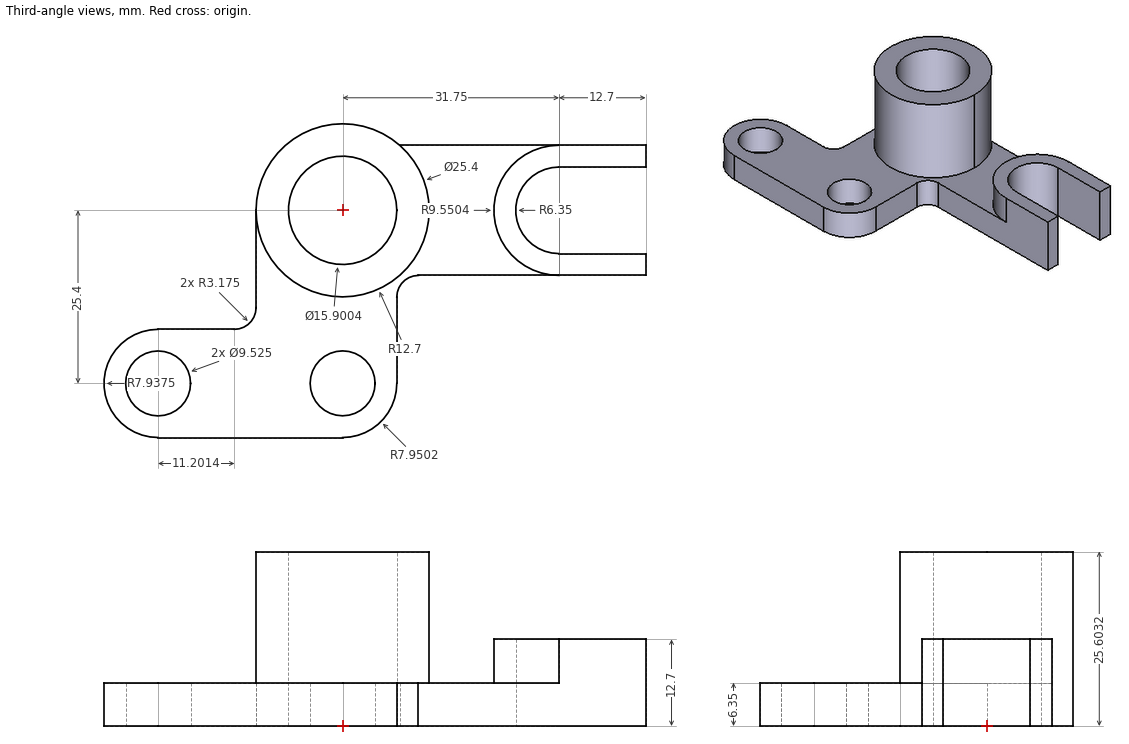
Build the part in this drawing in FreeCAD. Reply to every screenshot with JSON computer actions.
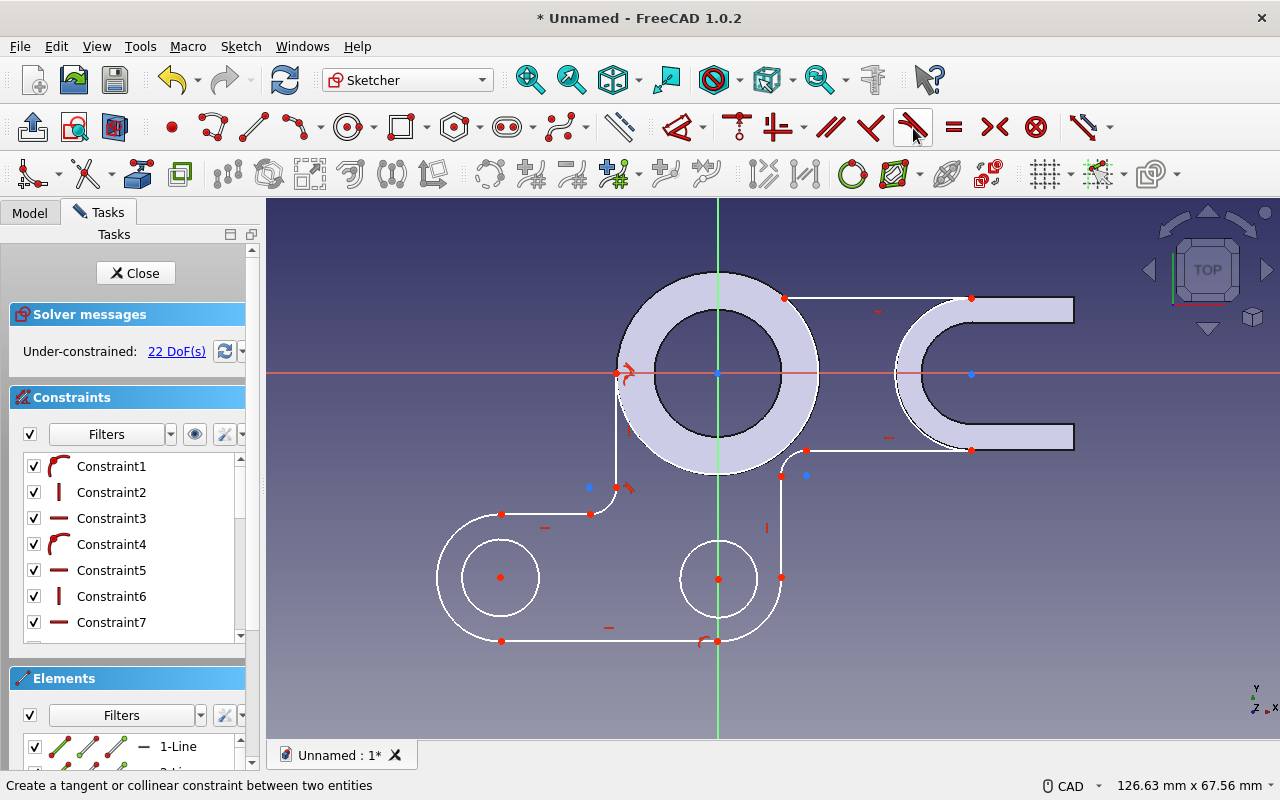
{"action": "left_click", "coordinate": [564, 514]}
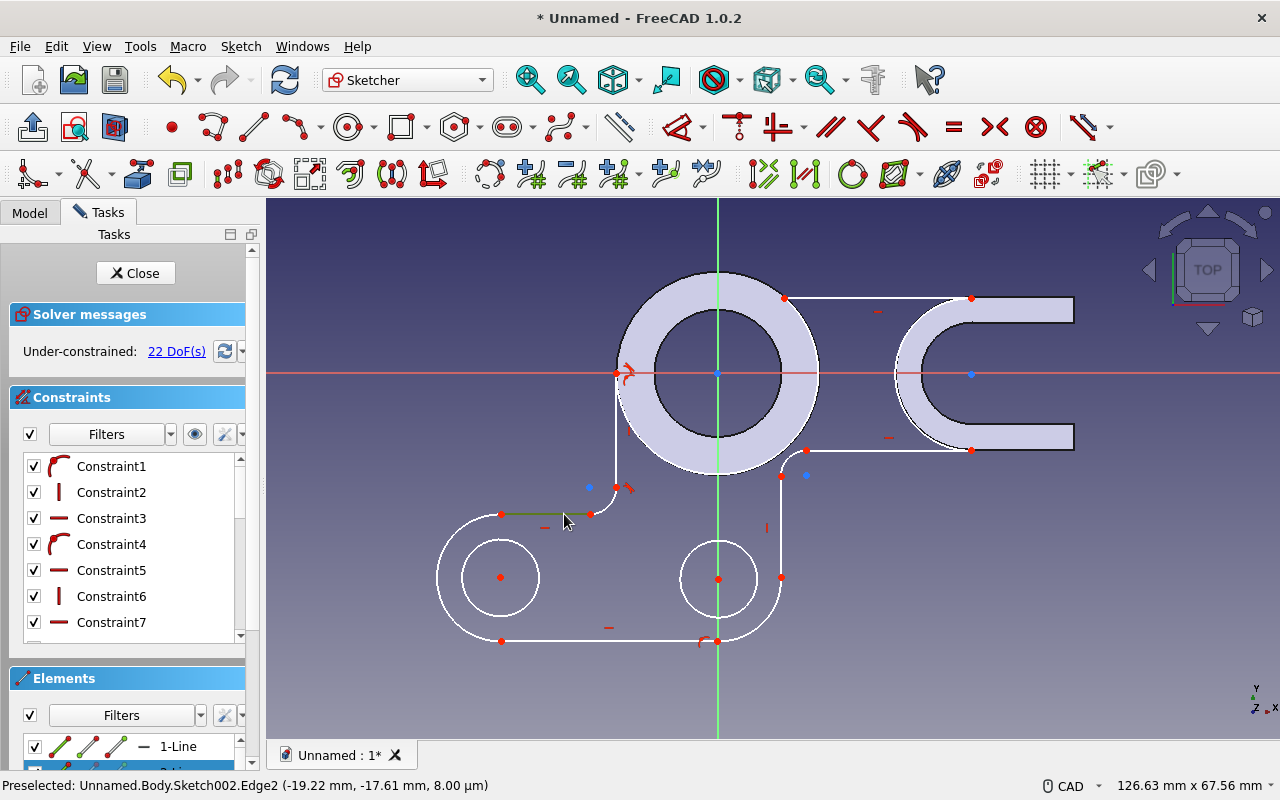
{"action": "left_click", "coordinate": [602, 511]}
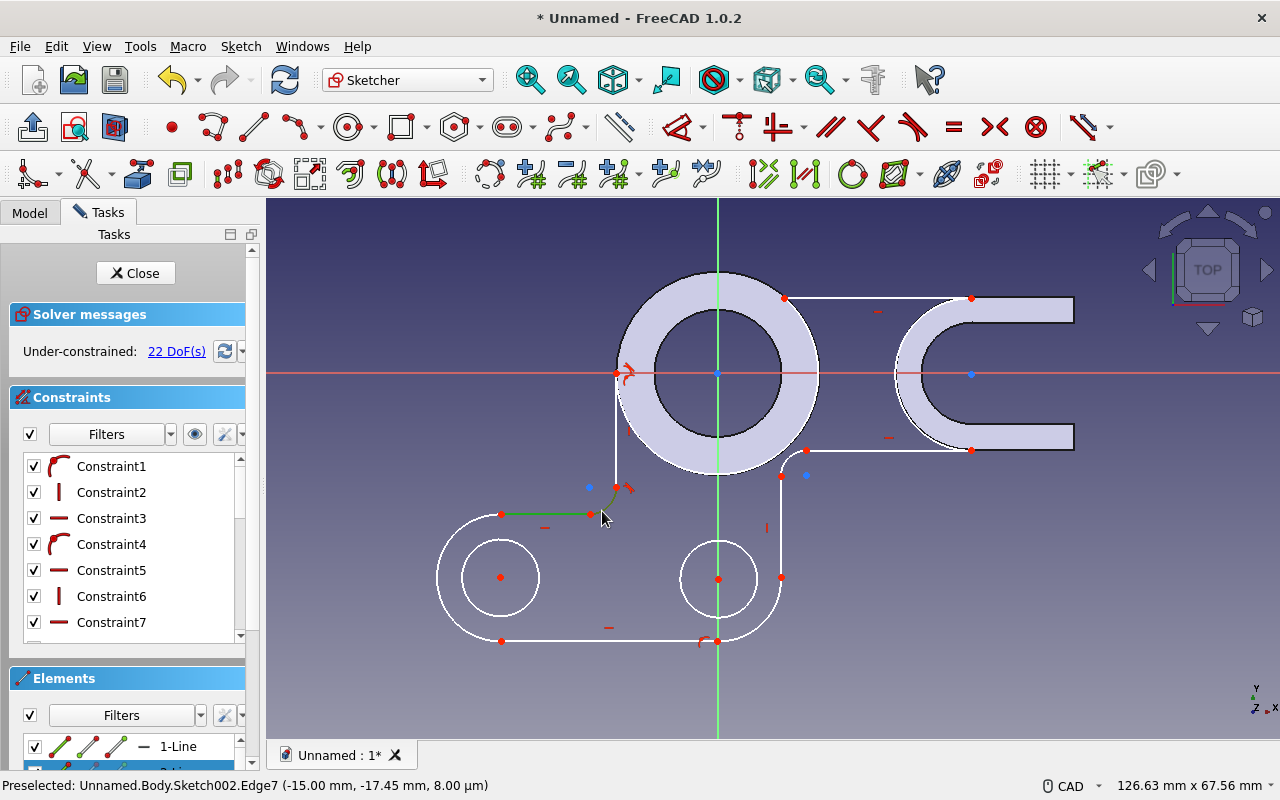
{"action": "left_click", "coordinate": [913, 128]}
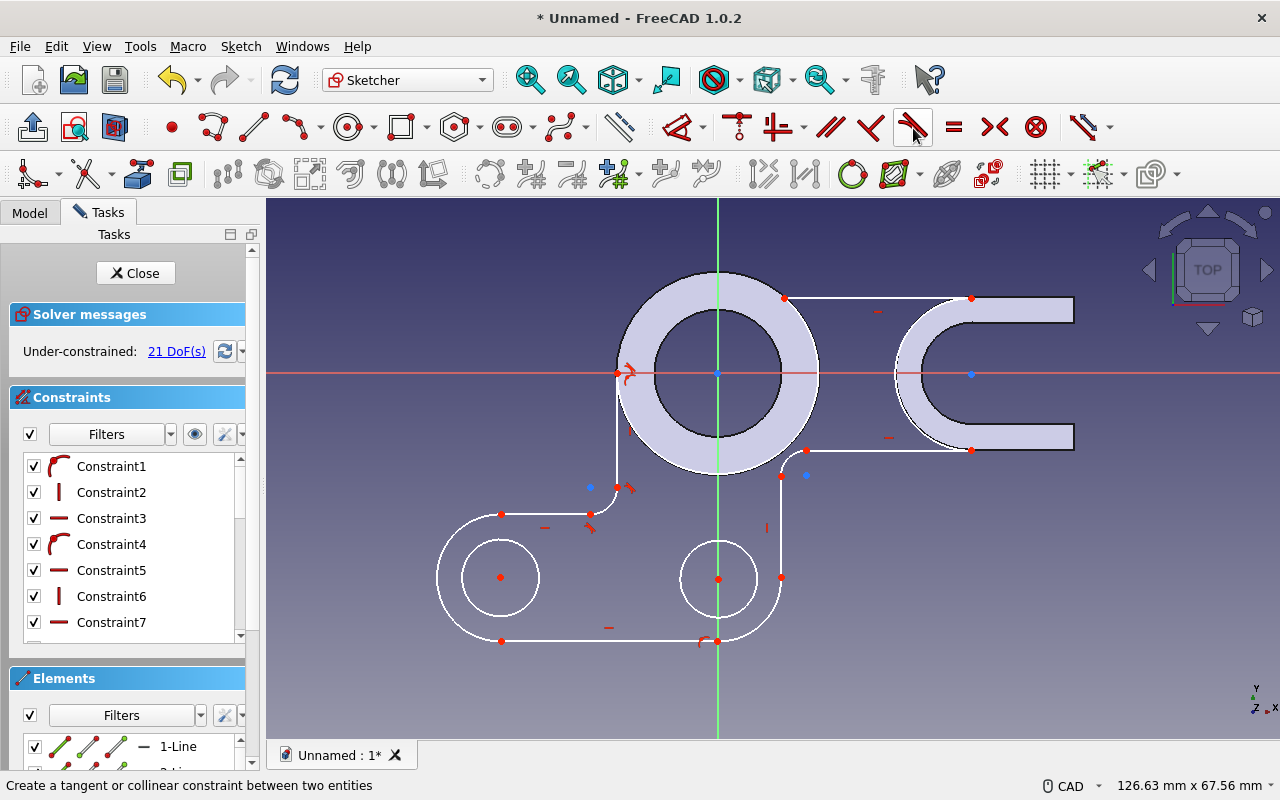
{"action": "left_click", "coordinate": [564, 514]}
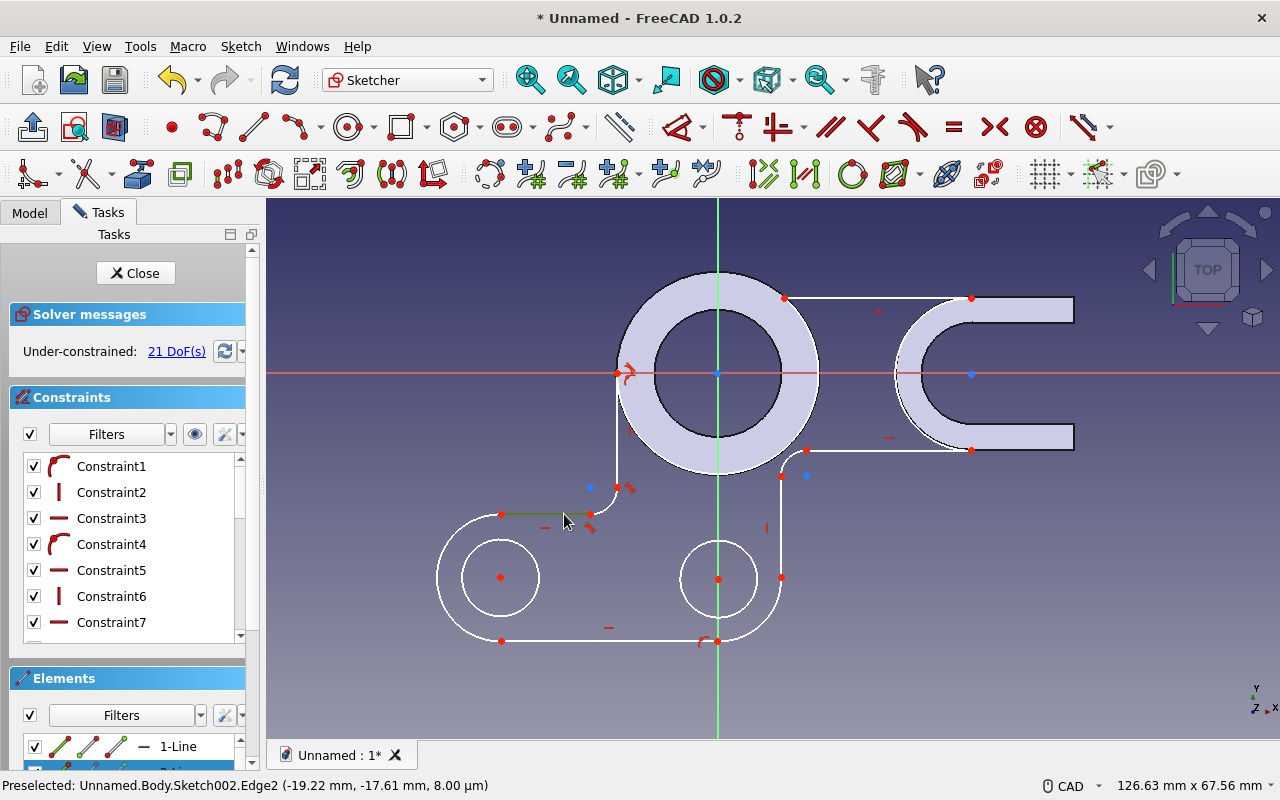
{"action": "left_click", "coordinate": [449, 540]}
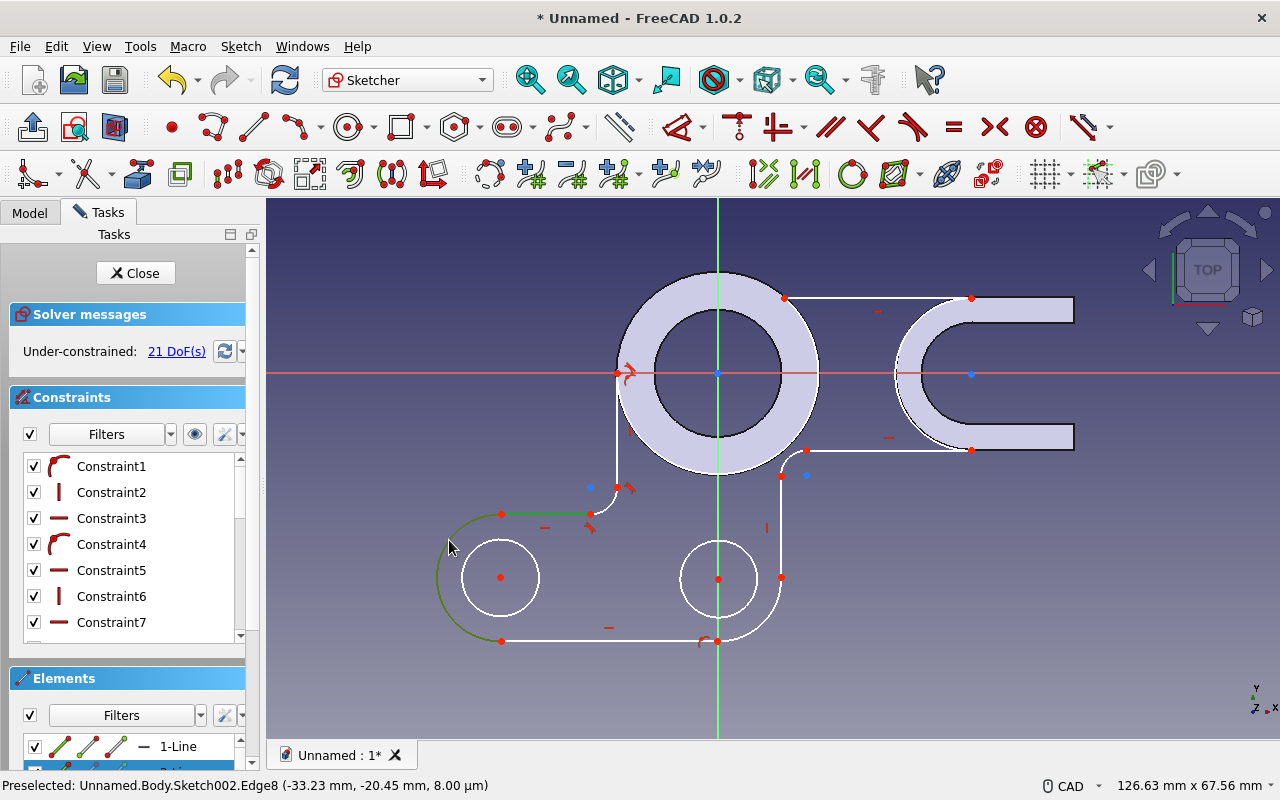
{"action": "left_click", "coordinate": [913, 128]}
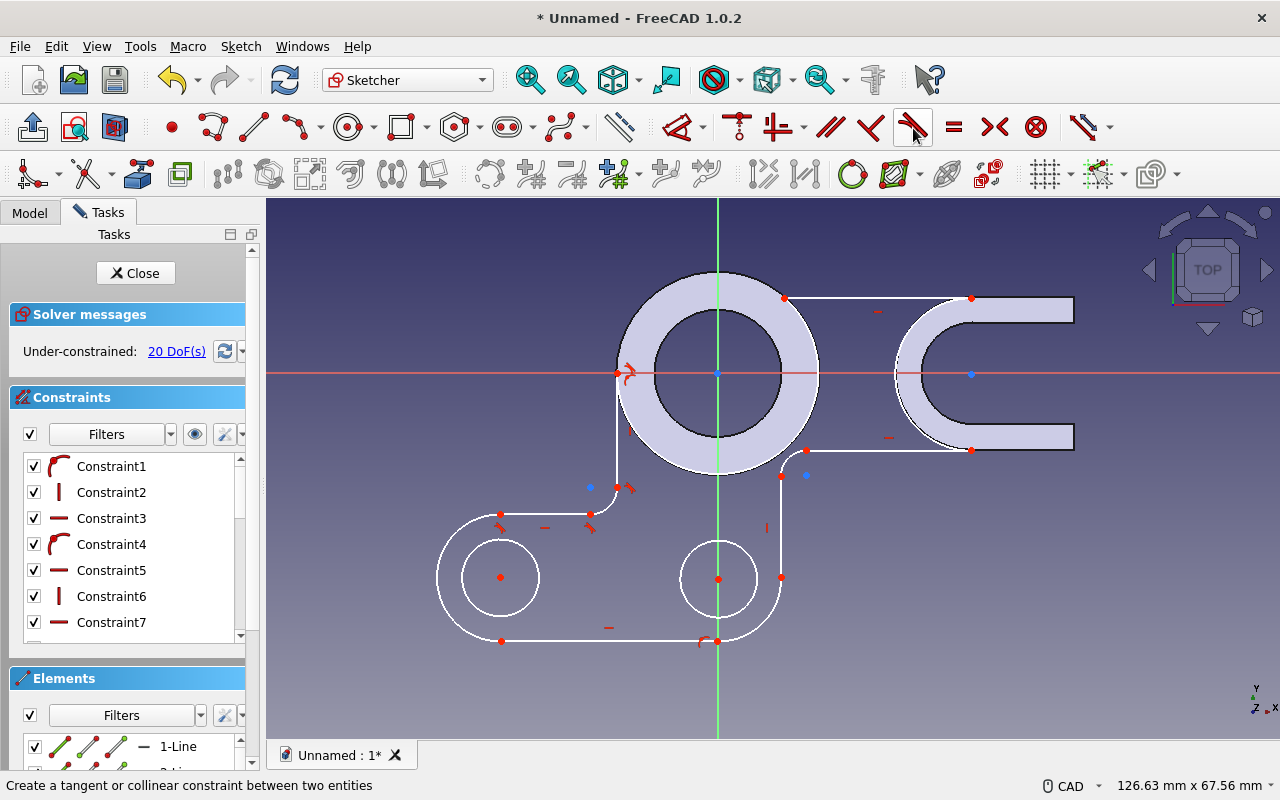
{"action": "left_click", "coordinate": [566, 641]}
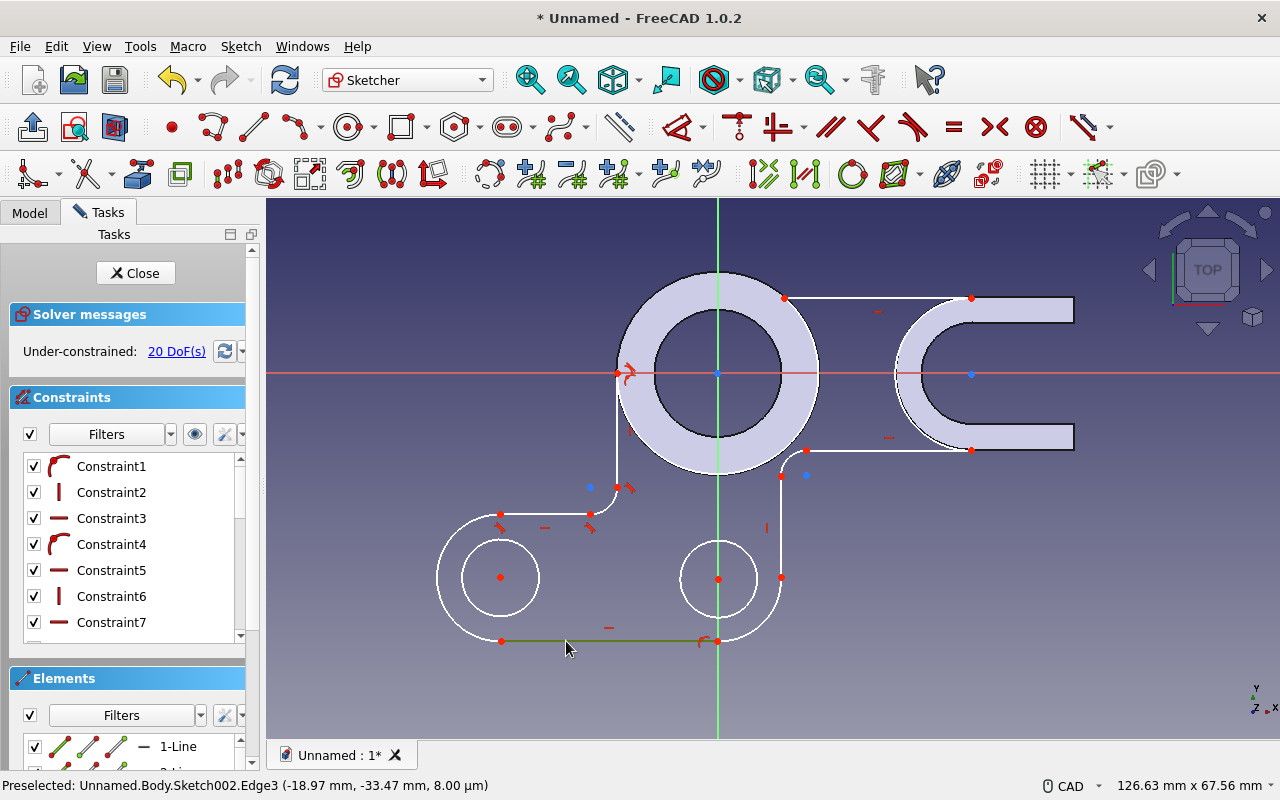
{"action": "left_click", "coordinate": [449, 541]}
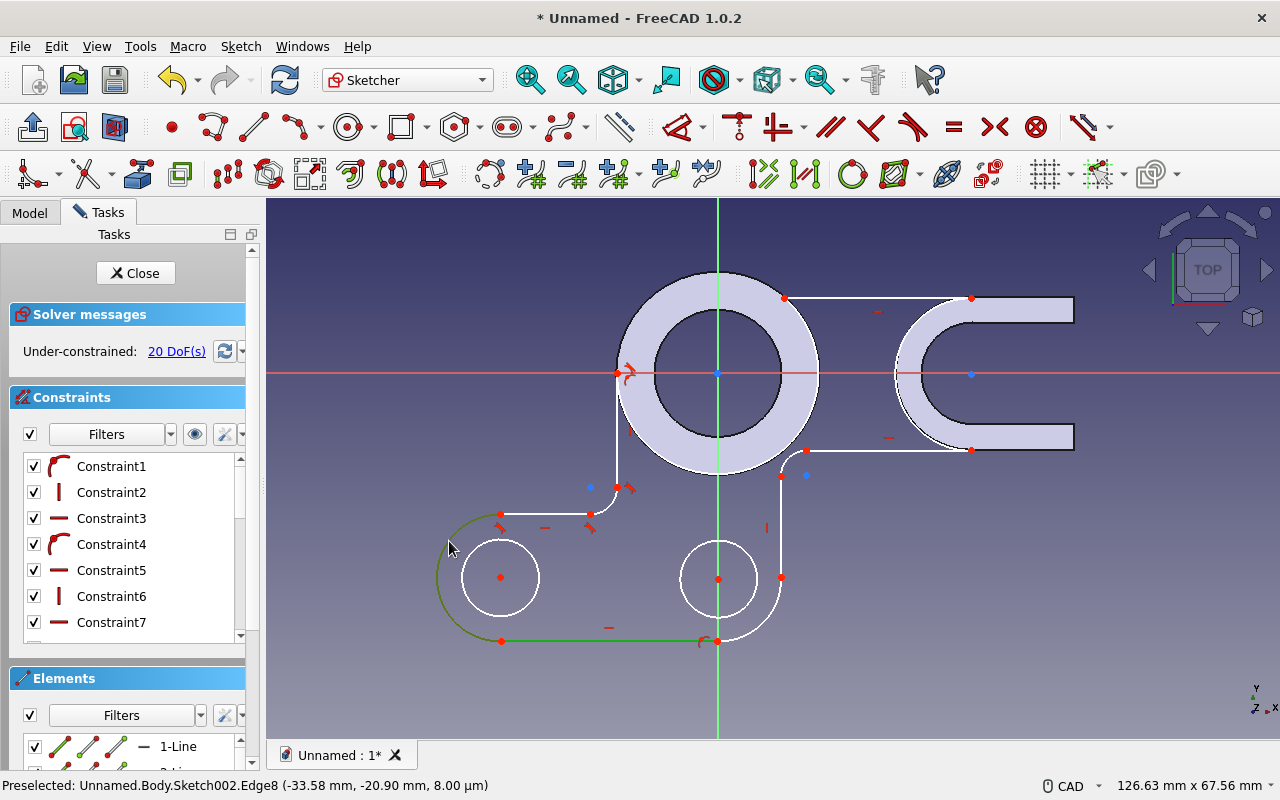
{"action": "left_click", "coordinate": [913, 128]}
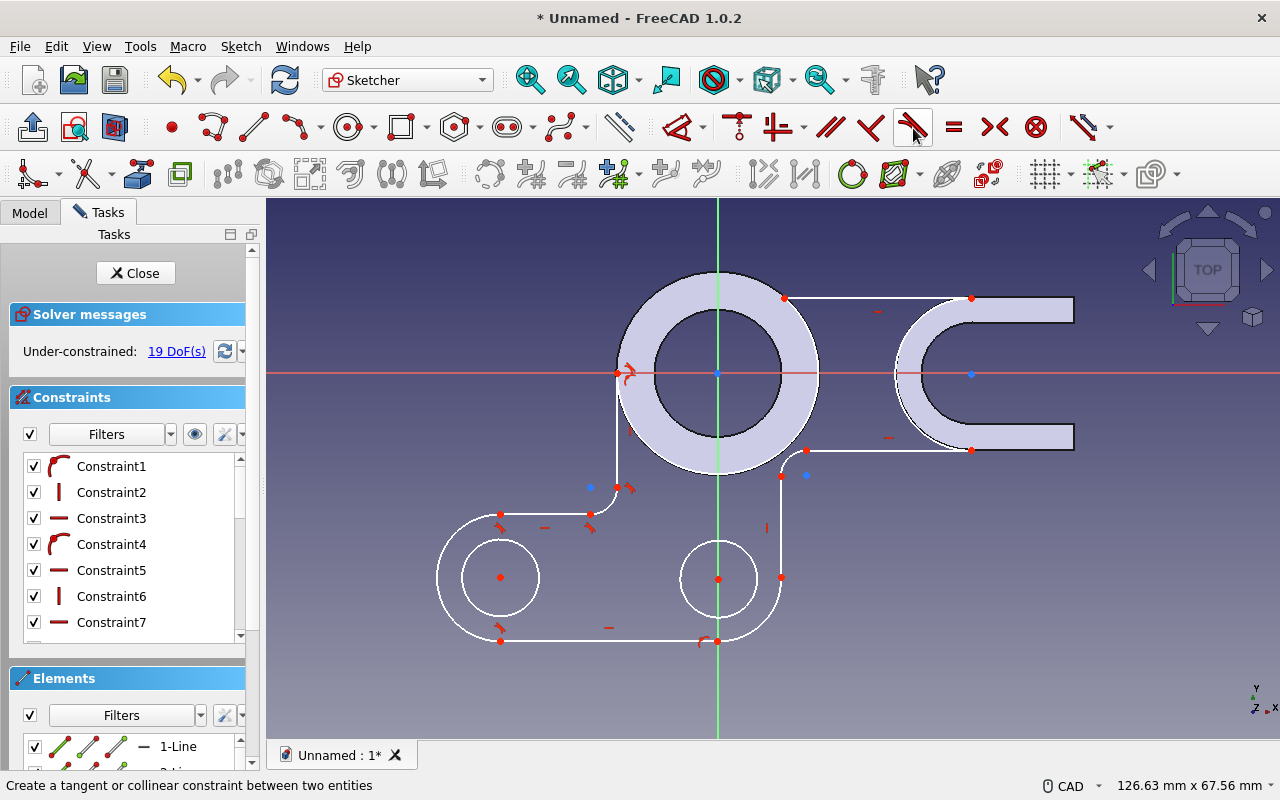
{"action": "left_click", "coordinate": [566, 641]}